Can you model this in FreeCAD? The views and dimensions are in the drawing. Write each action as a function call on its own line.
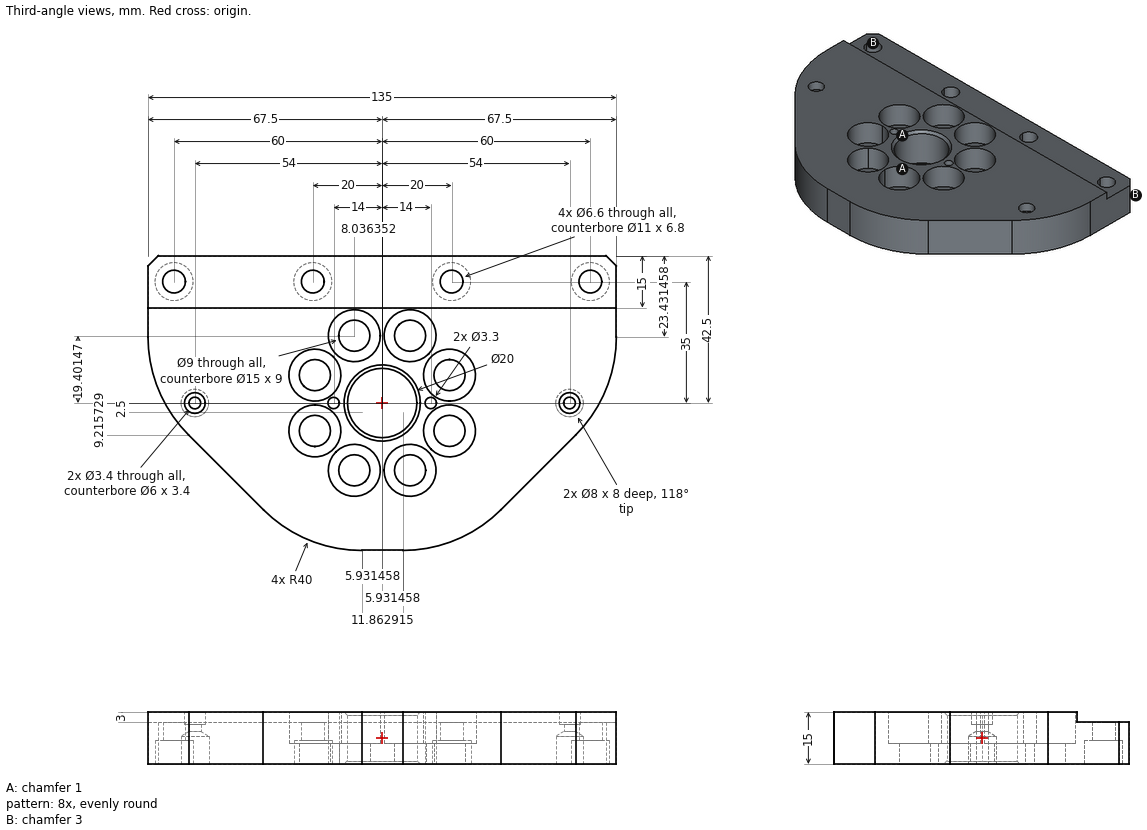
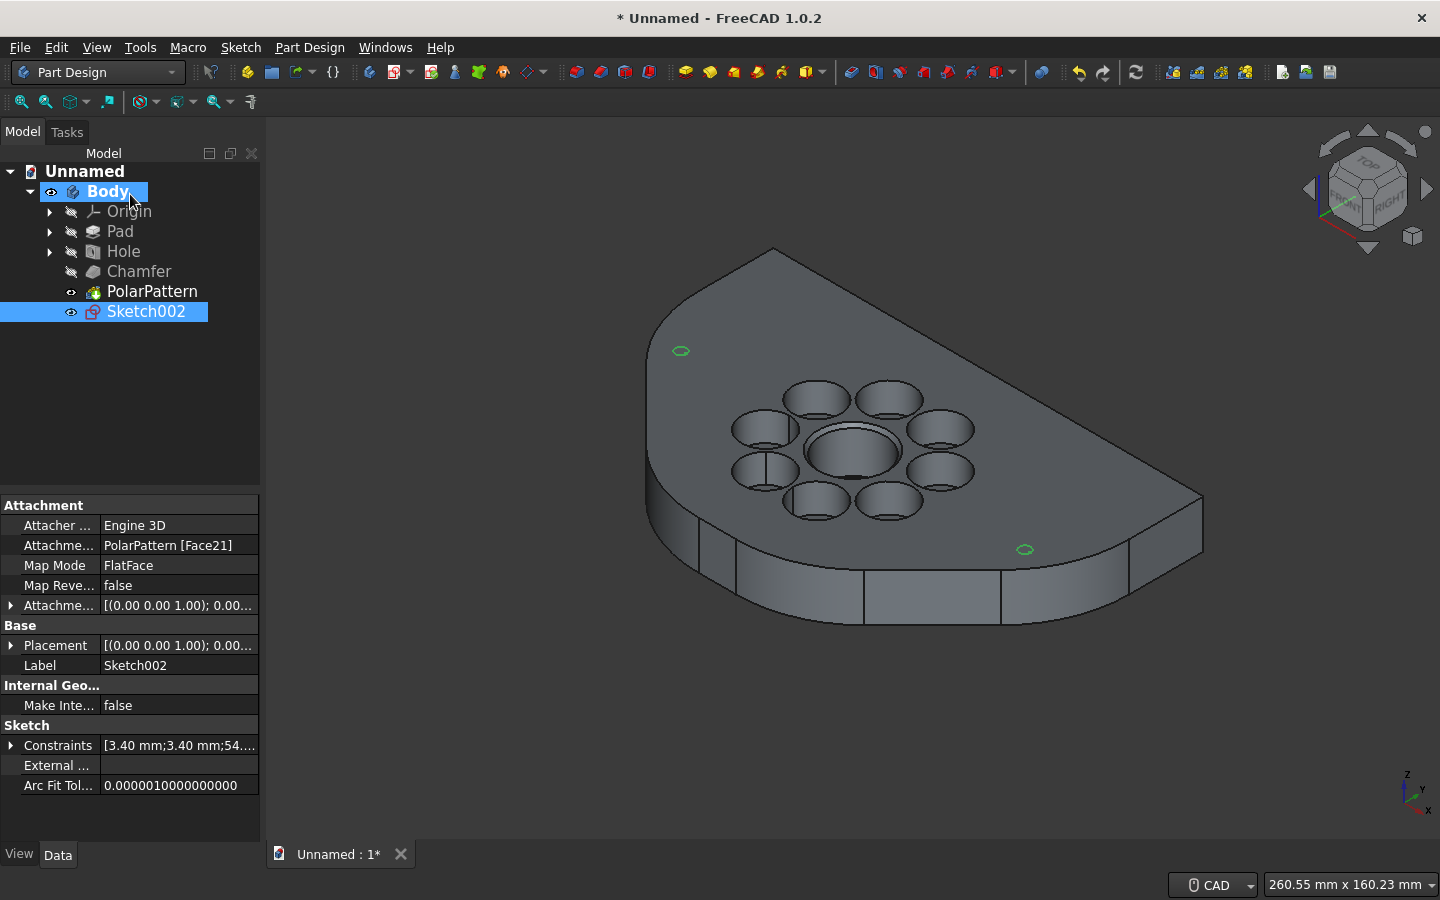
click(876, 72)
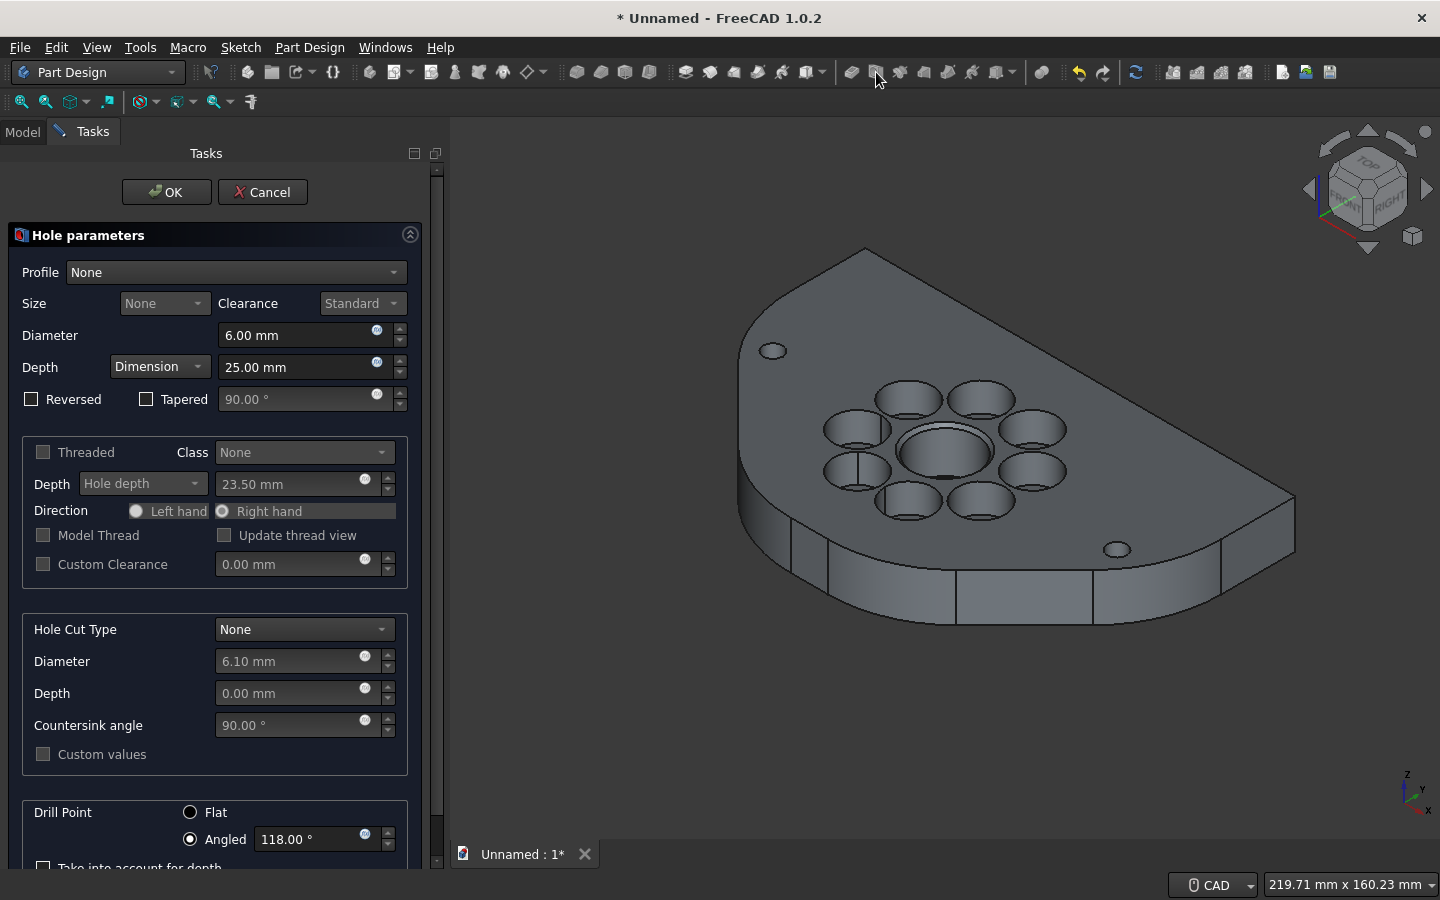
triple_click(305, 335)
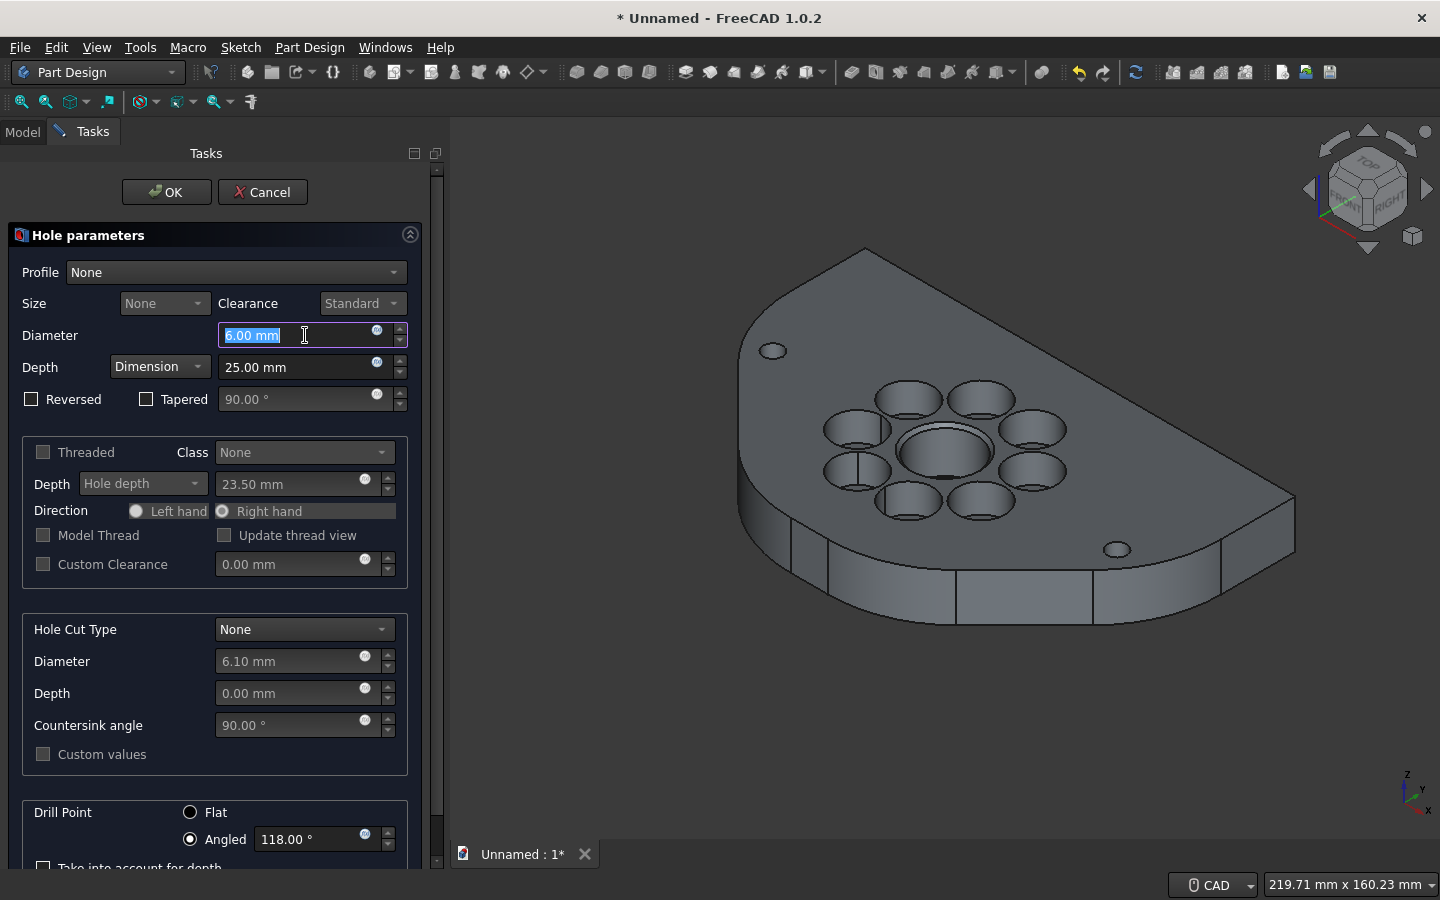
text(3.4)
key(Tab)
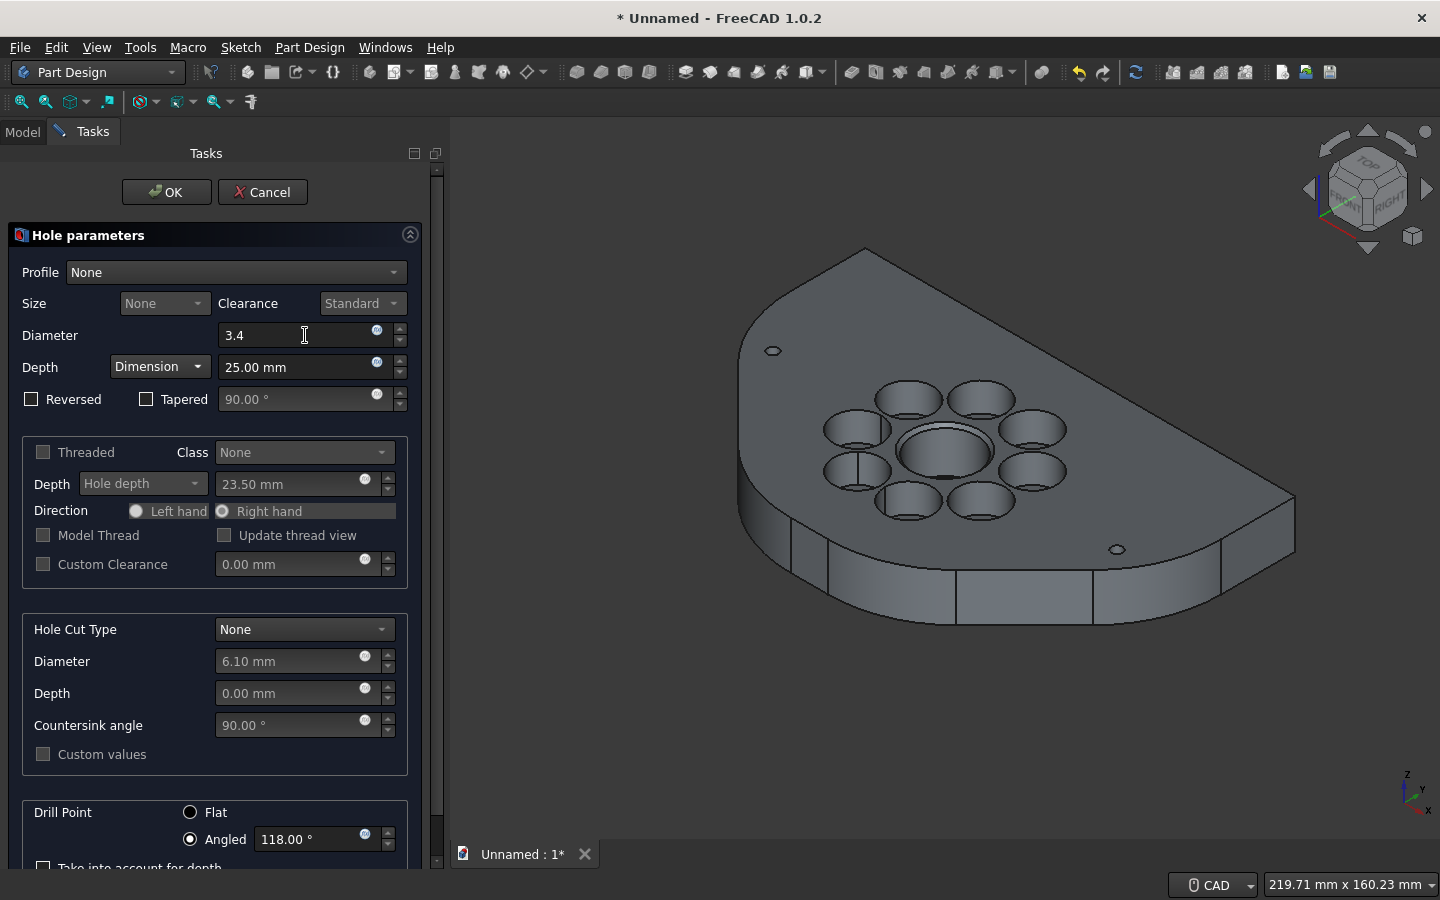
click(161, 366)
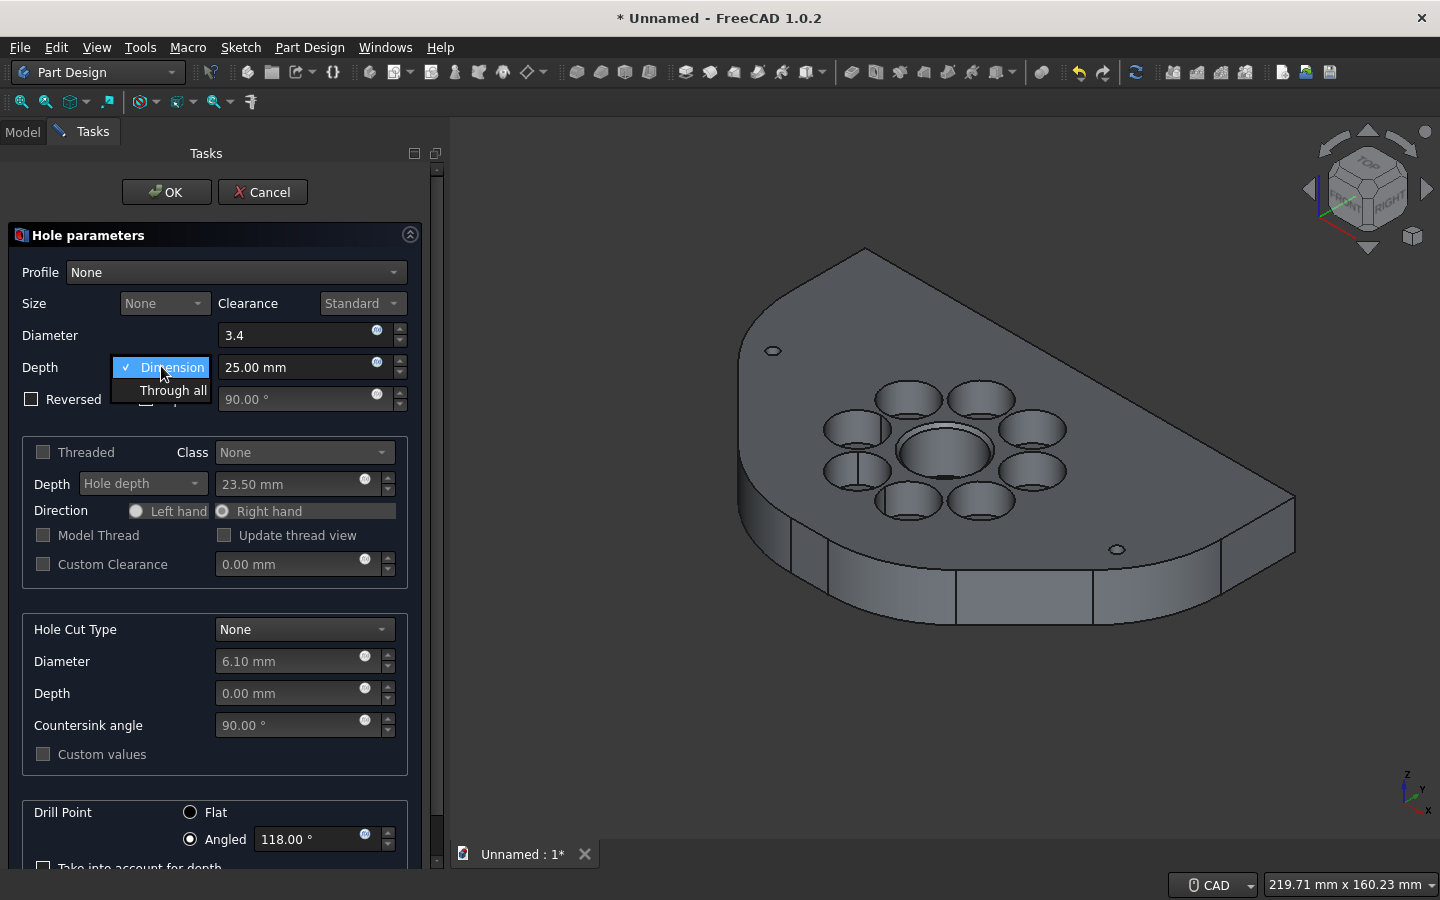
click(160, 390)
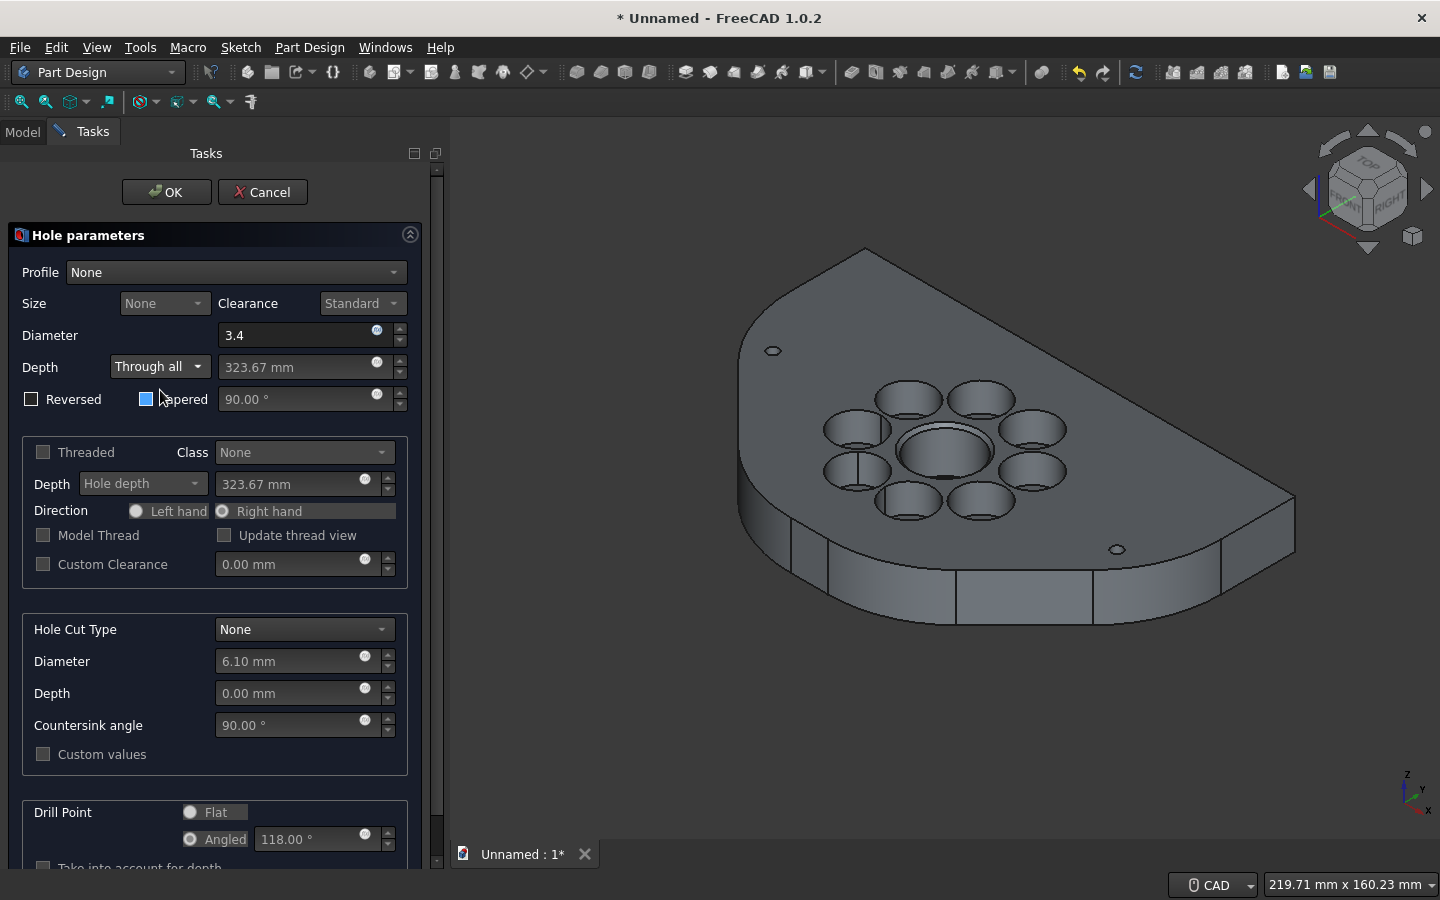
click(306, 630)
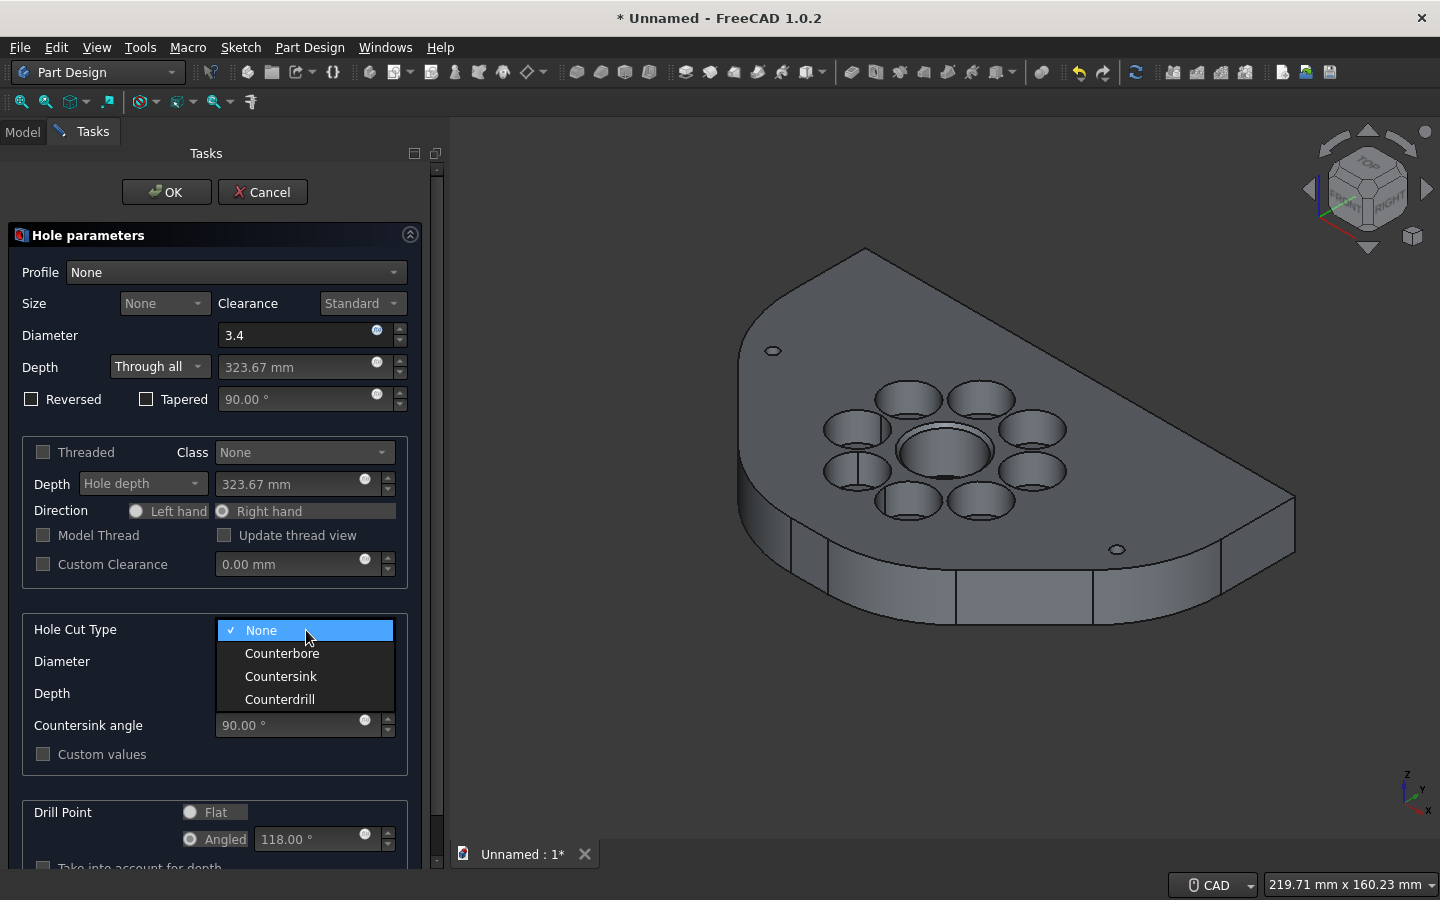
click(304, 654)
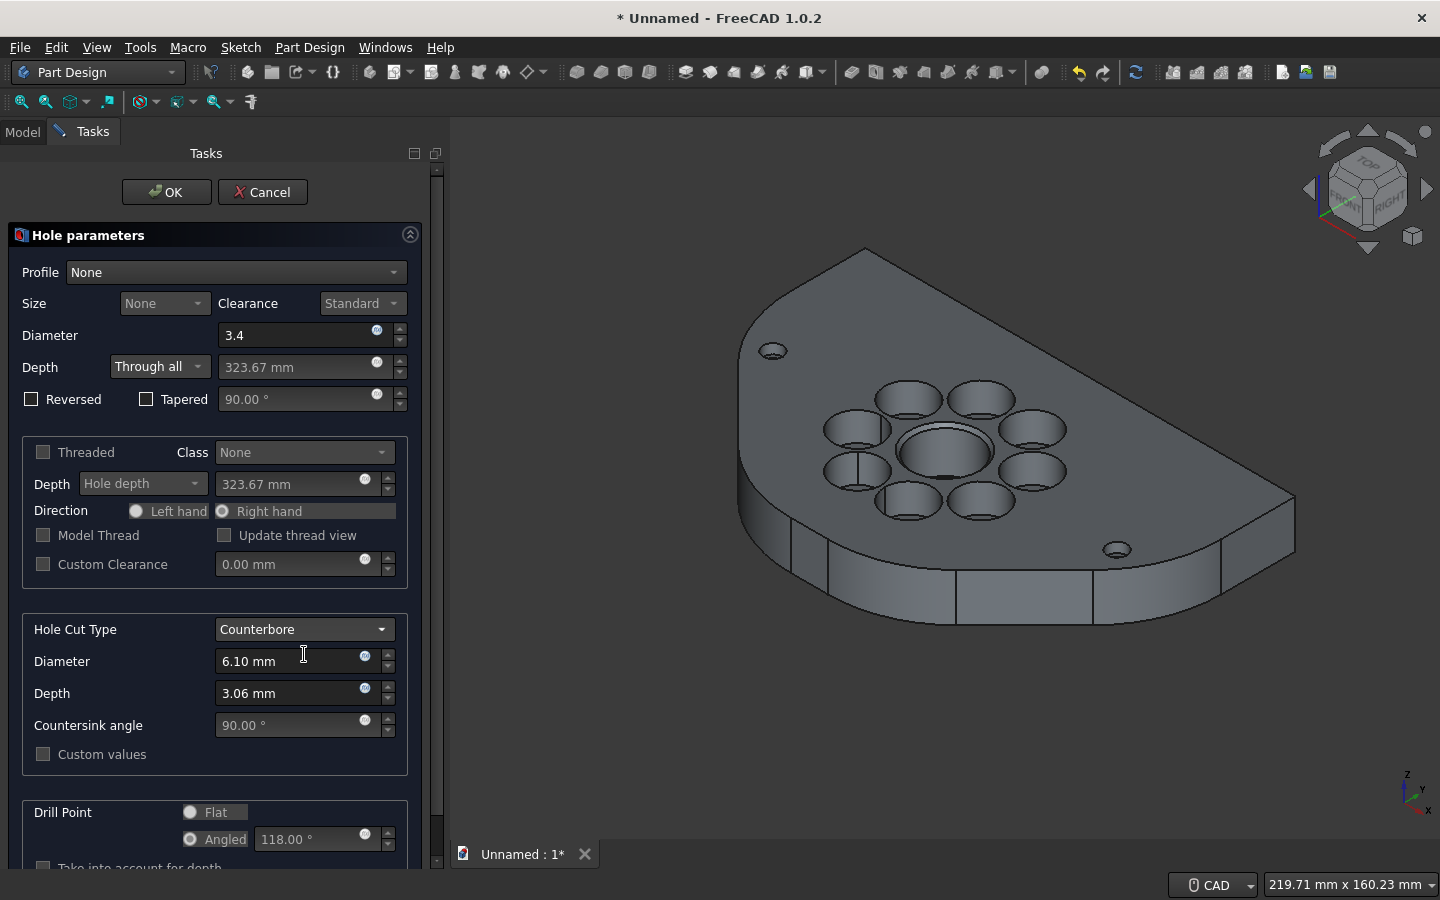
triple_click(298, 661)